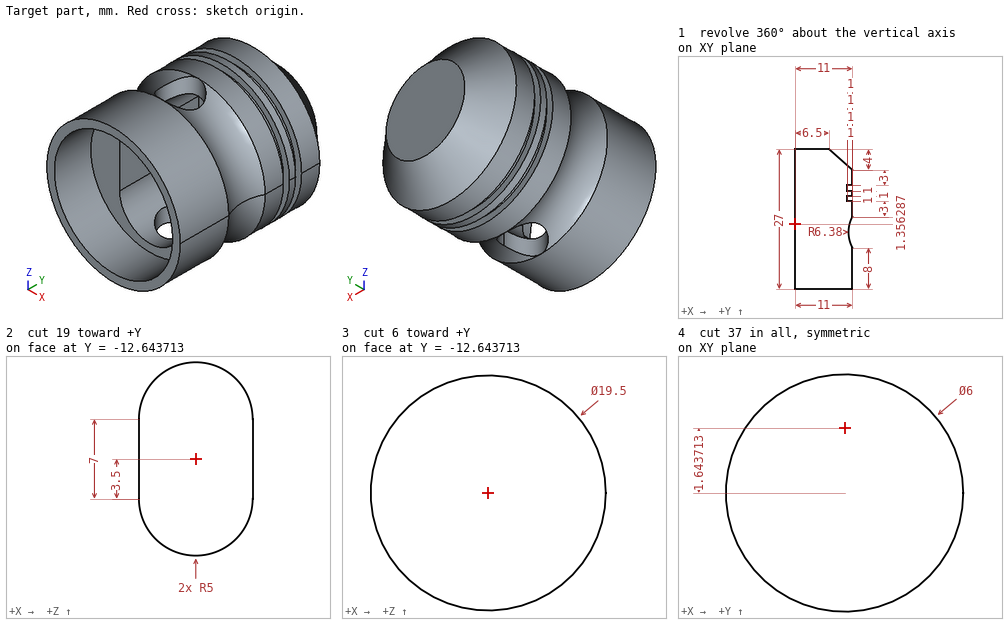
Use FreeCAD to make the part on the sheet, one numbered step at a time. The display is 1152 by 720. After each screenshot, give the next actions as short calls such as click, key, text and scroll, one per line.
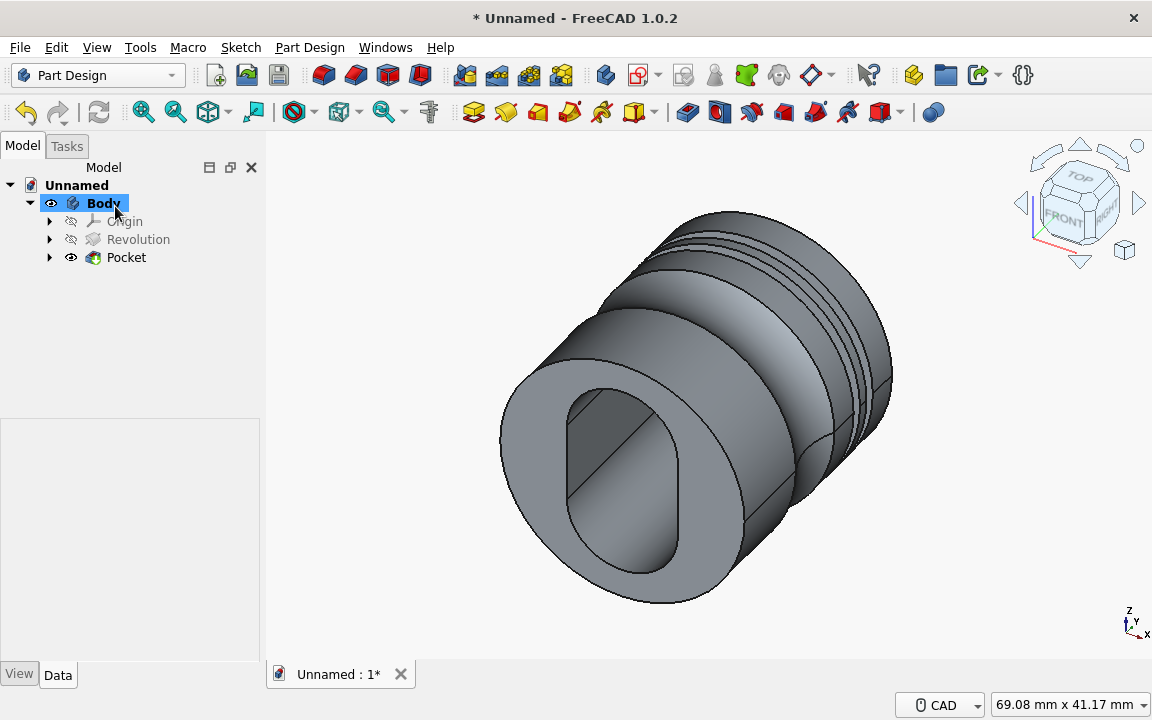
click(692, 569)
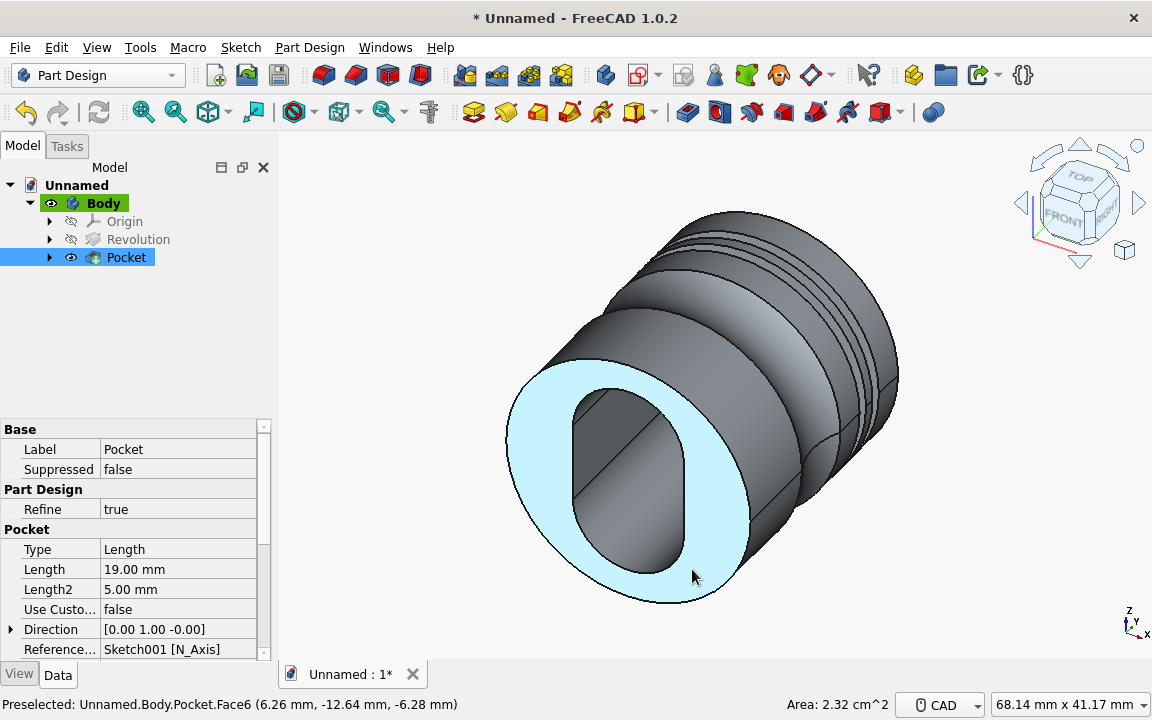
click(638, 76)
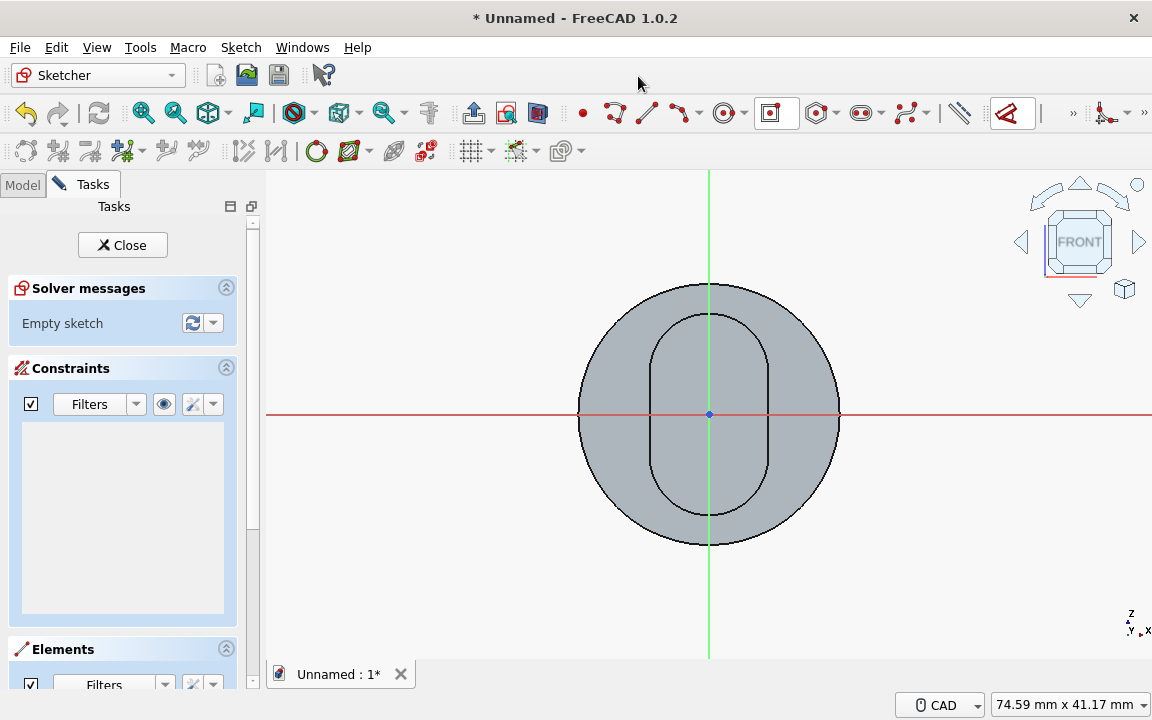
click(724, 114)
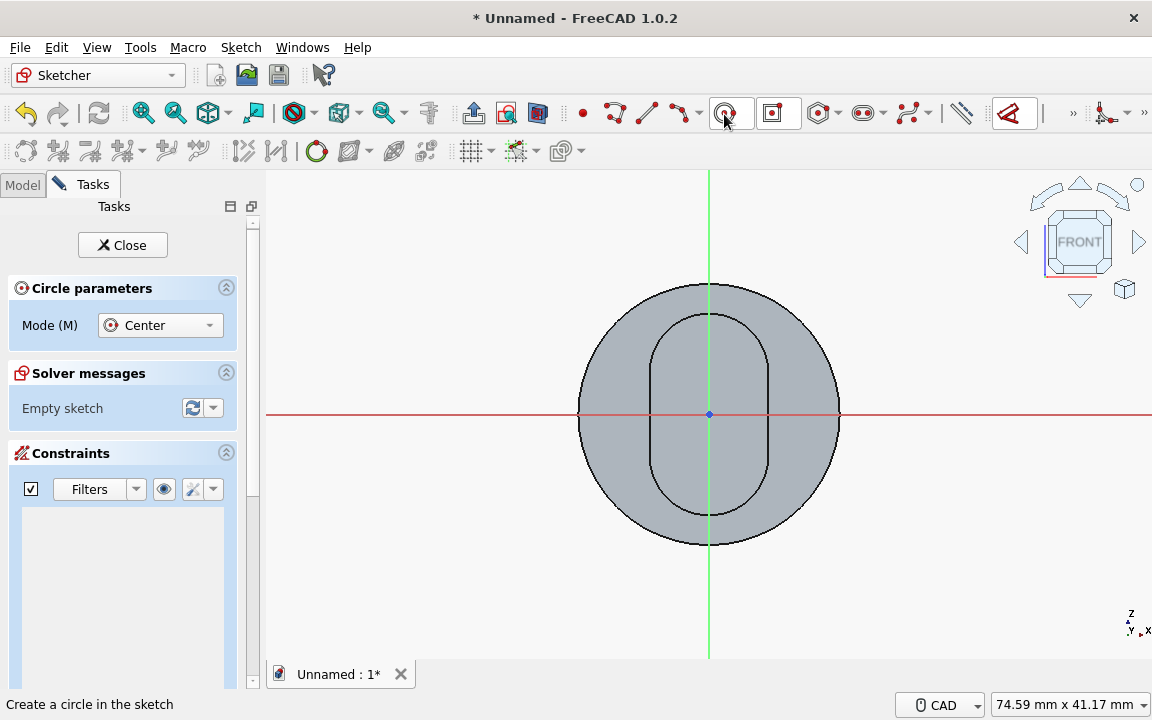
click(709, 415)
move(791, 333)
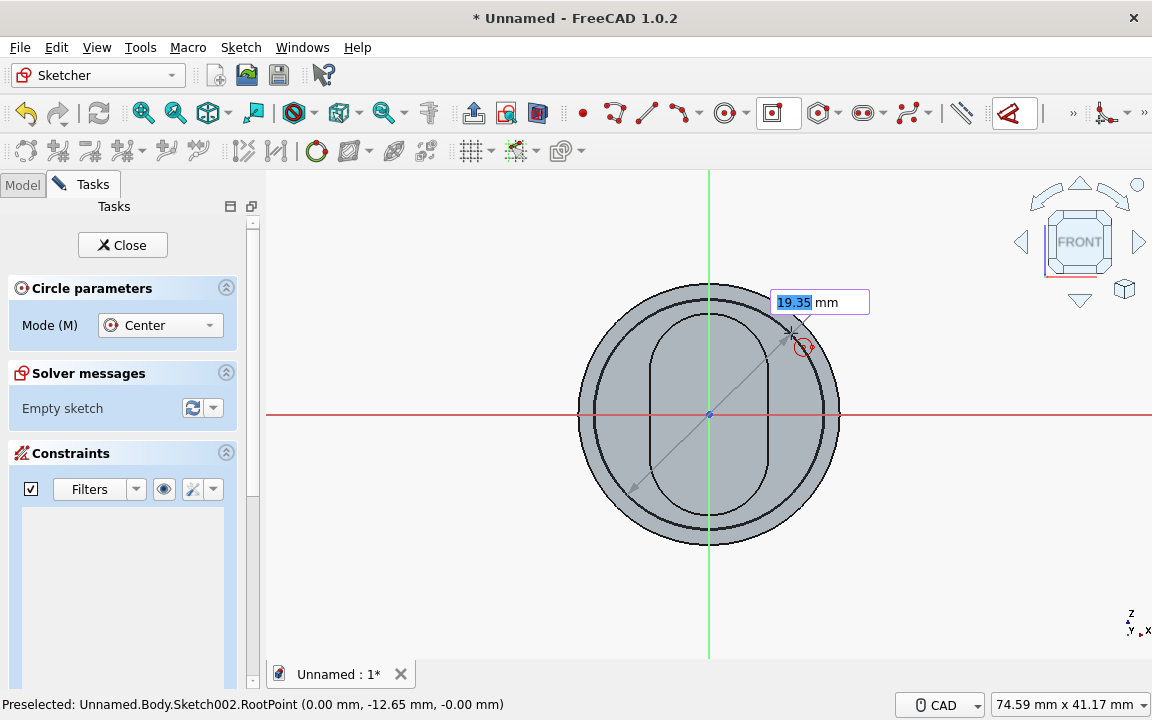
text(19.5)
key(Return)
key(Escape)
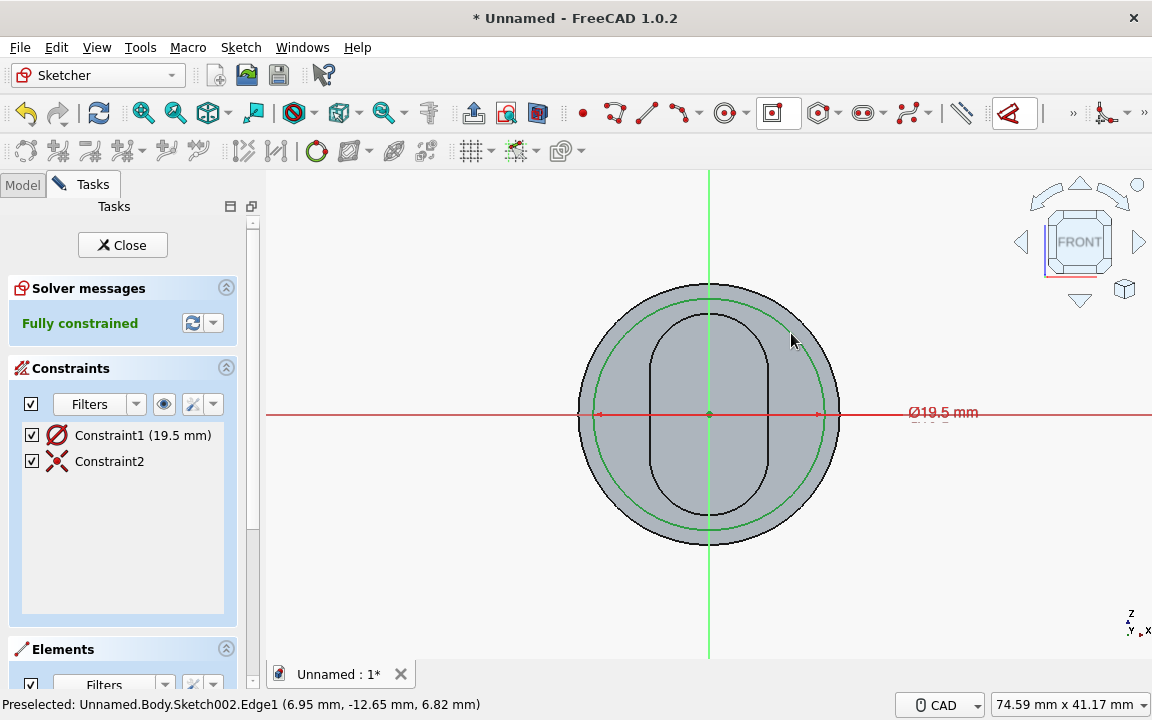
click(123, 245)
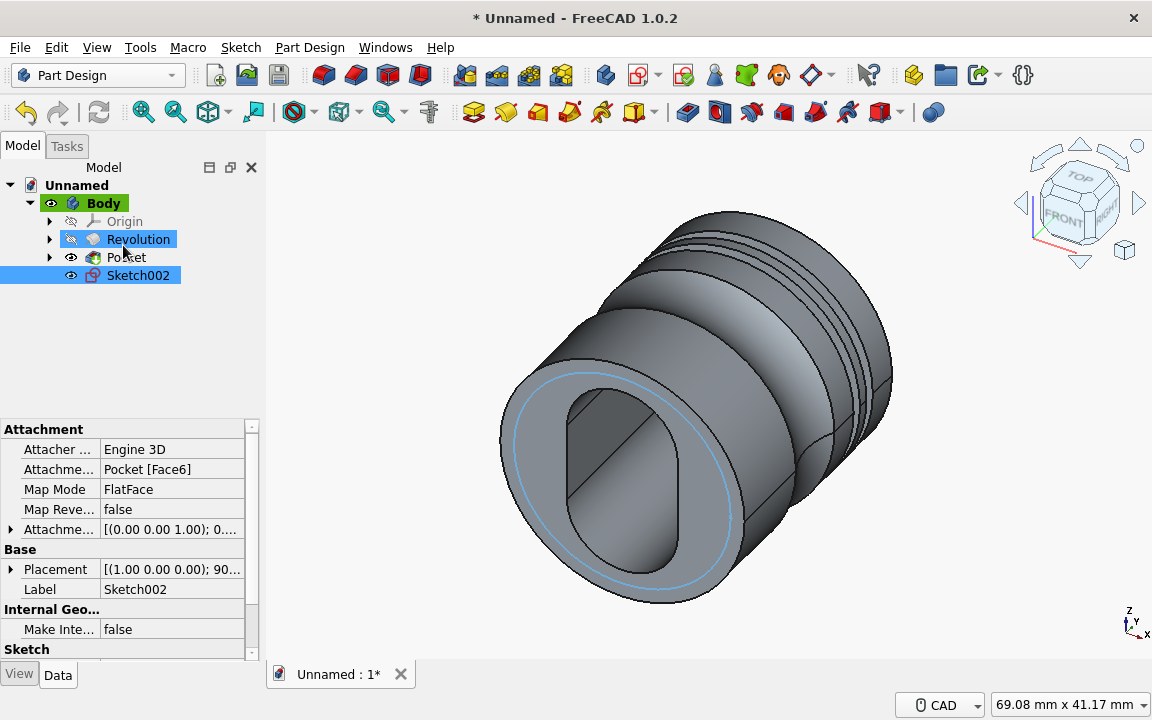
click(688, 112)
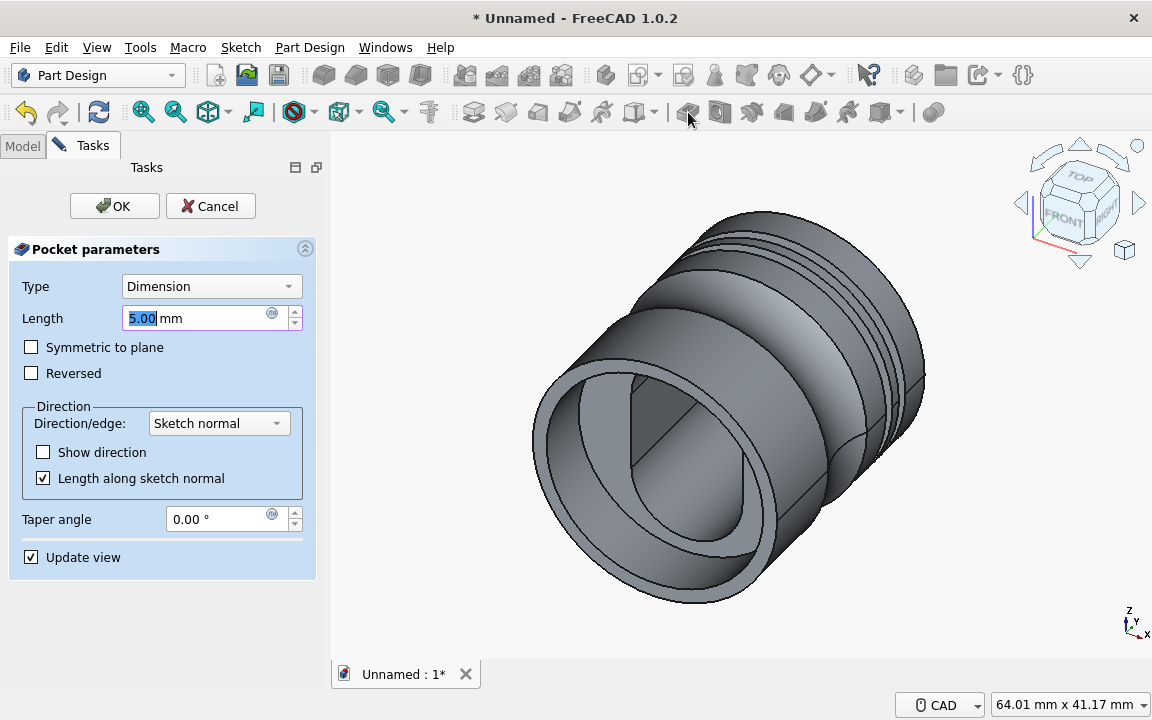
text(6)
key(Tab)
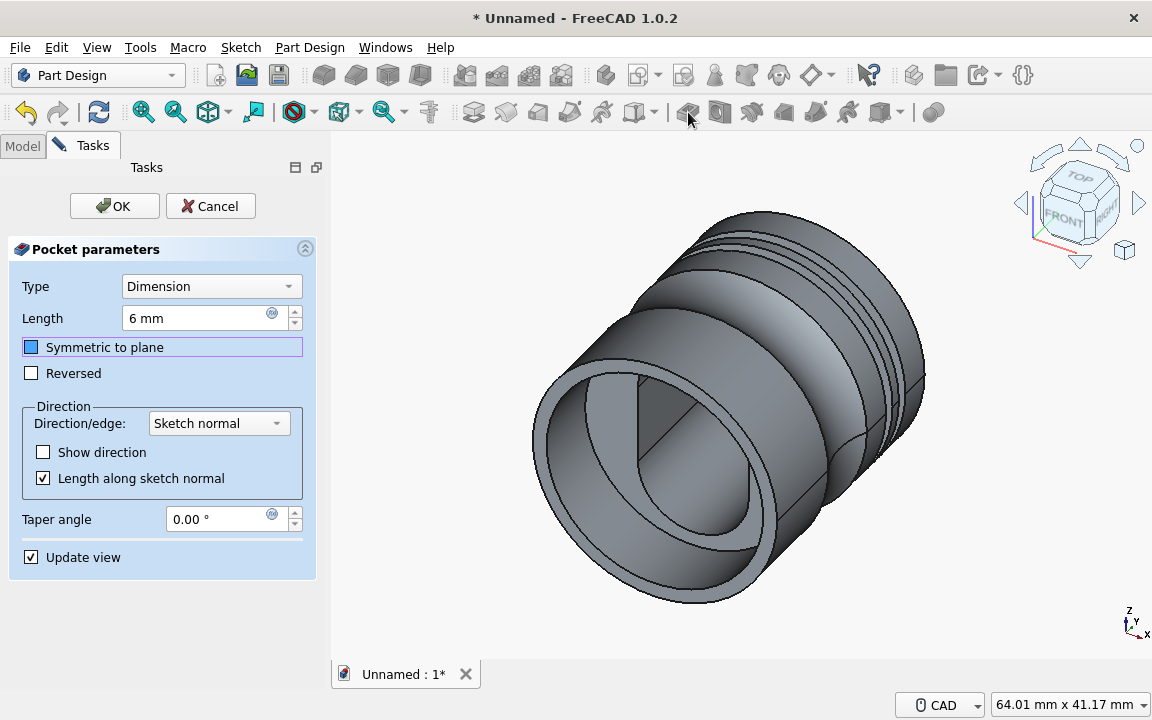
click(115, 206)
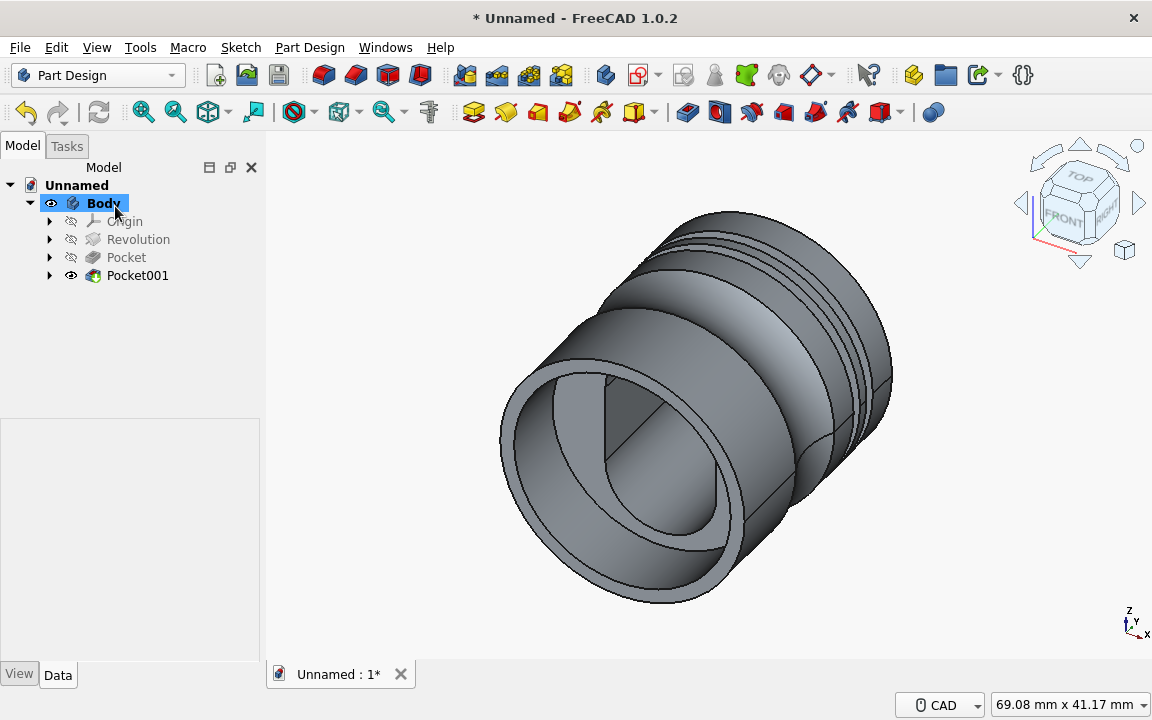
click(638, 76)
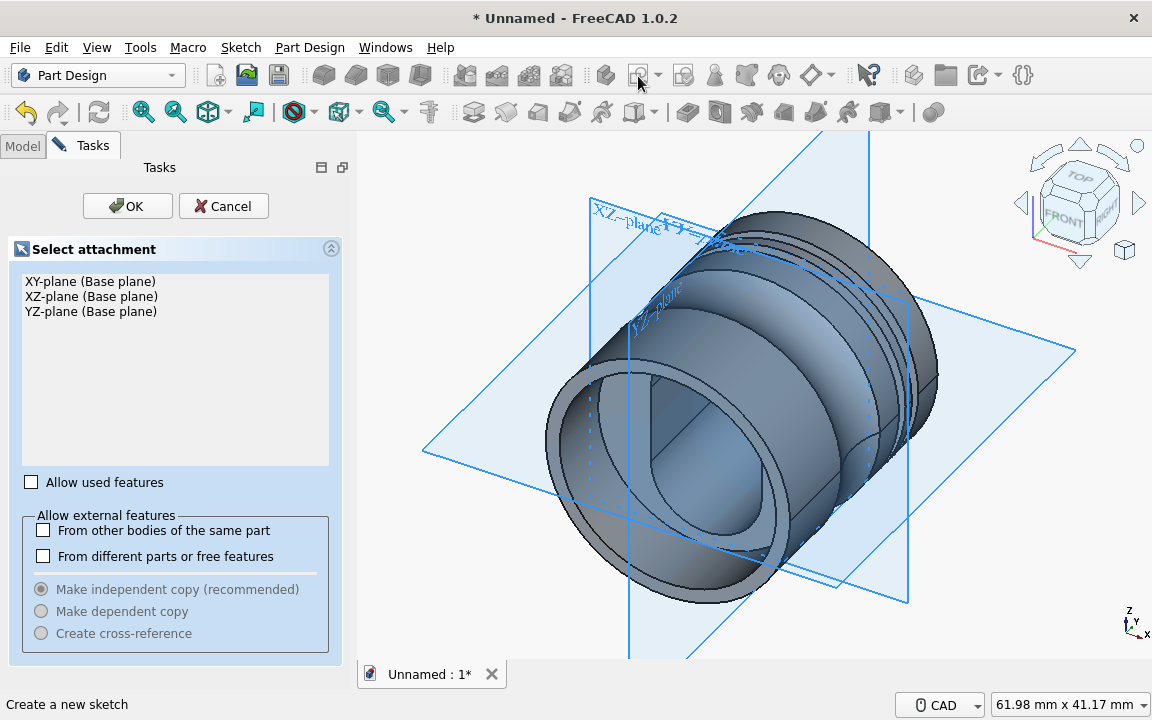
click(82, 282)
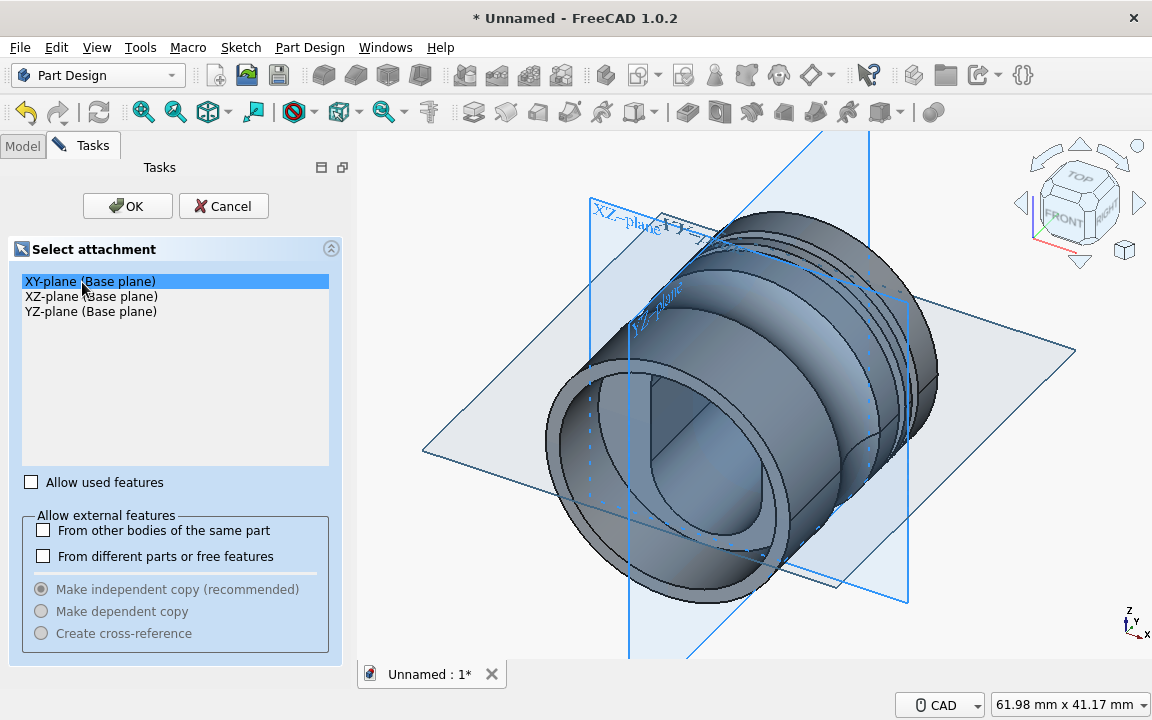
click(128, 206)